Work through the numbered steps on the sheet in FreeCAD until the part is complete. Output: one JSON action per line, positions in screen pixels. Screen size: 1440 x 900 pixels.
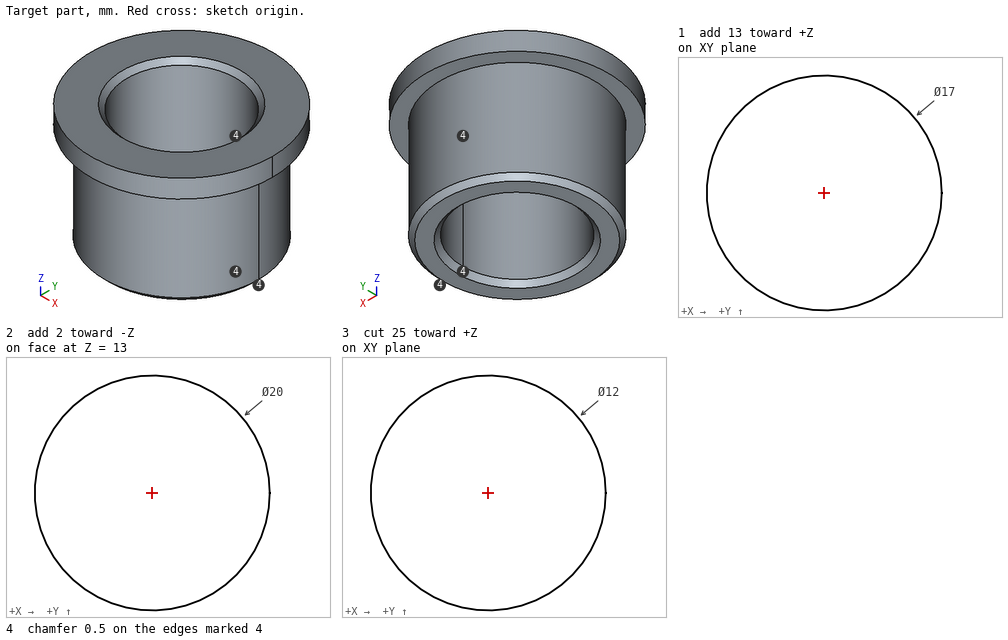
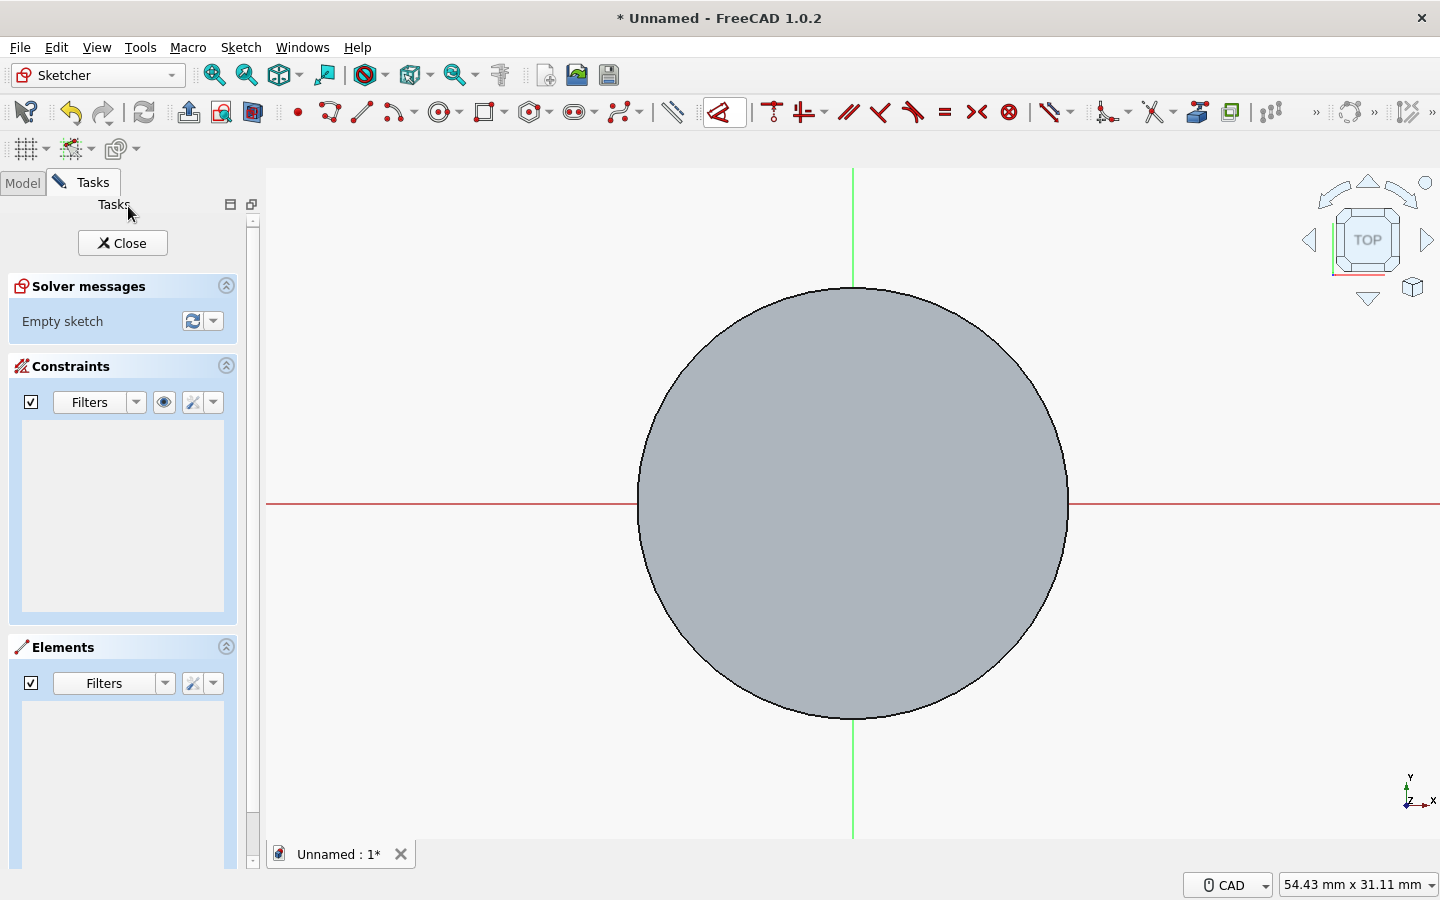
{"action": "key", "text": "q s"}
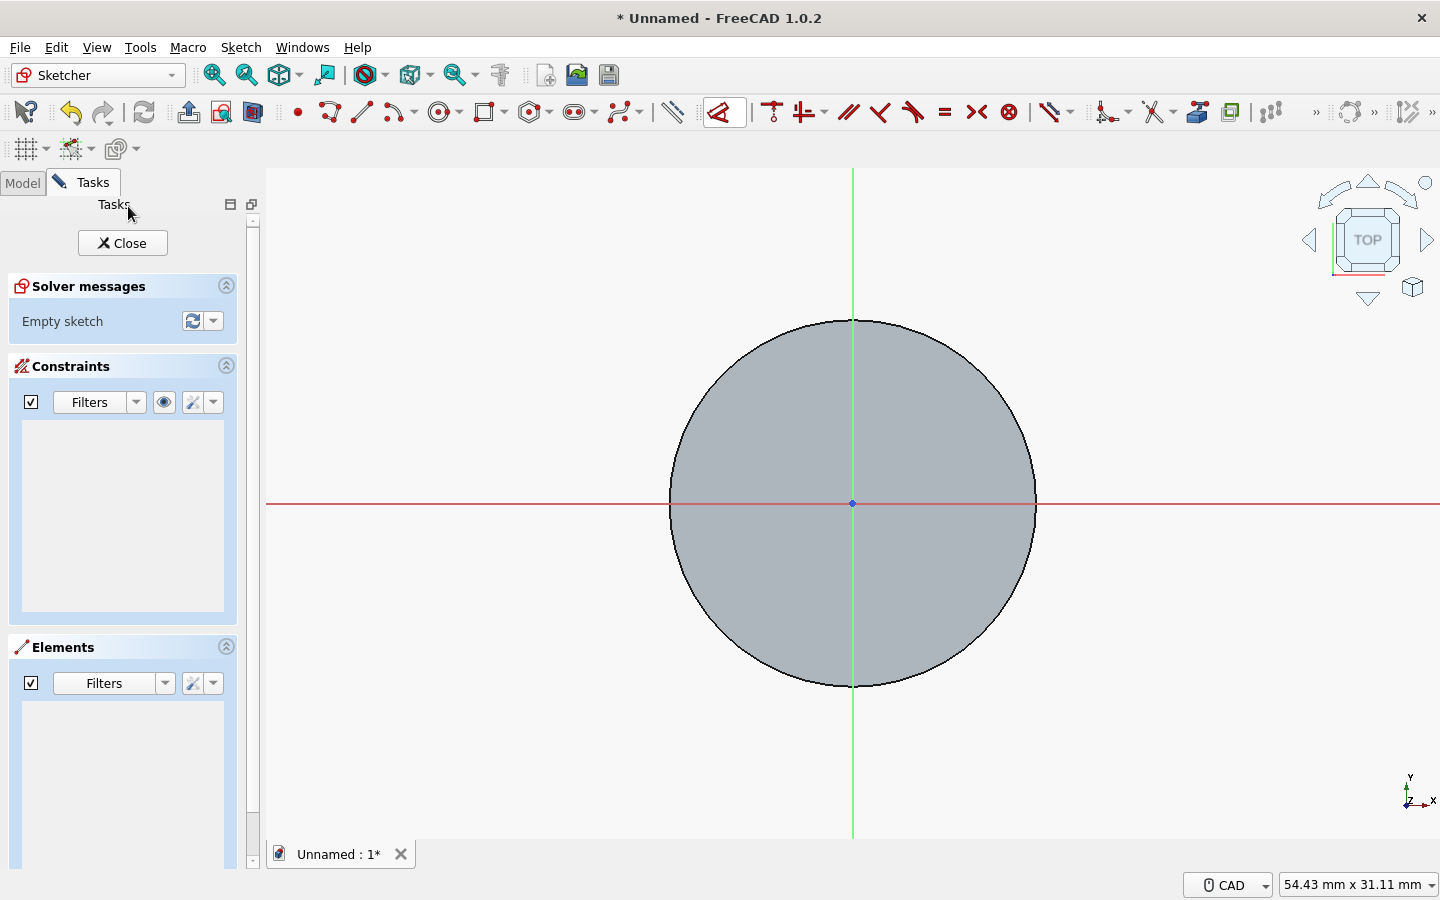
{"action": "scroll", "coordinate": [936, 504], "scroll_direction": "up", "scroll_amount": 3}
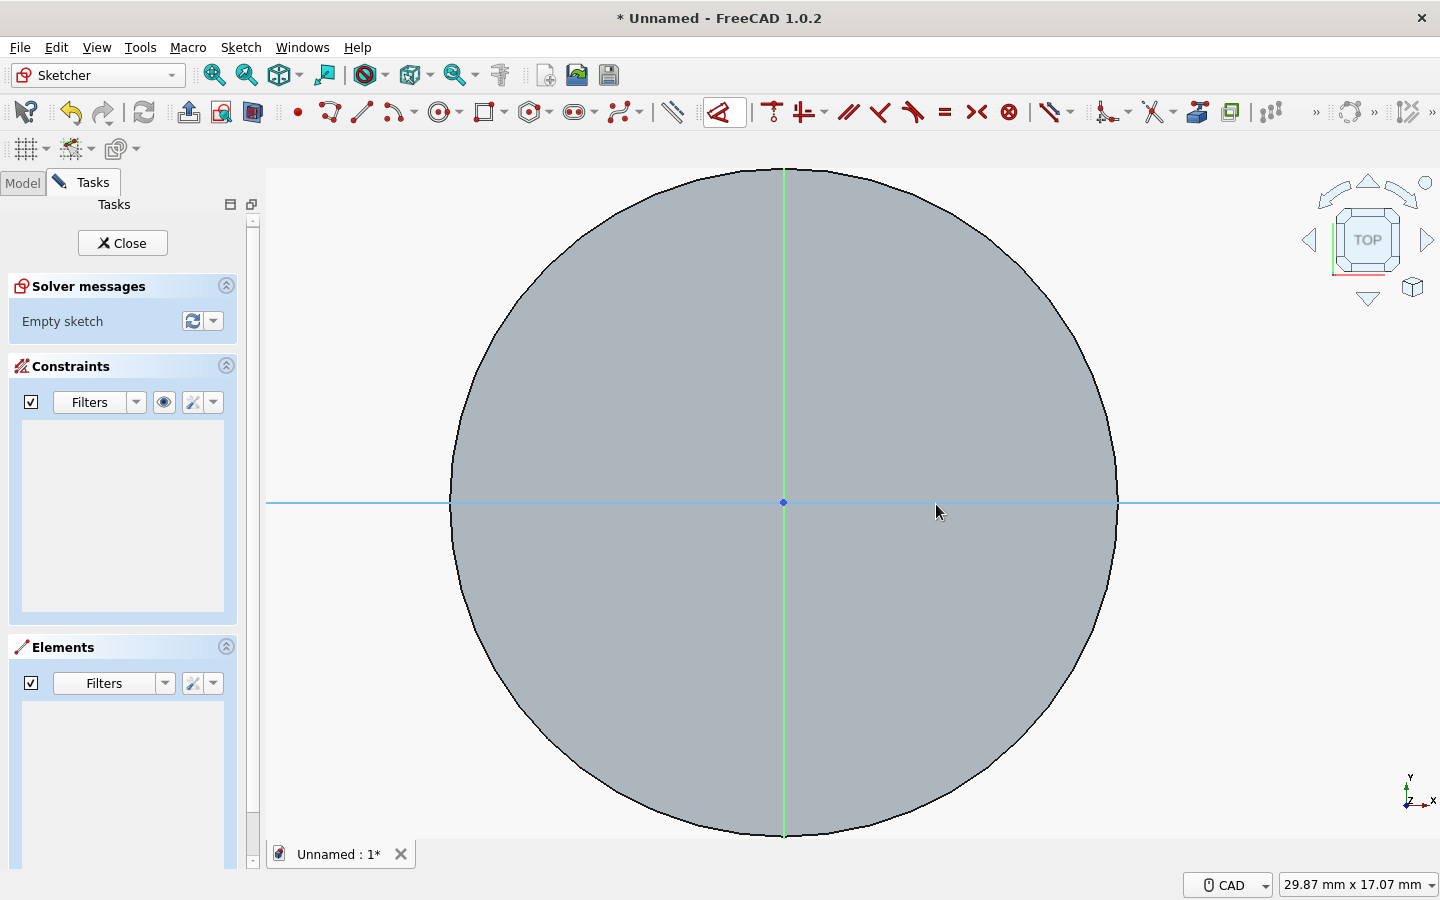
{"action": "key", "text": "g c"}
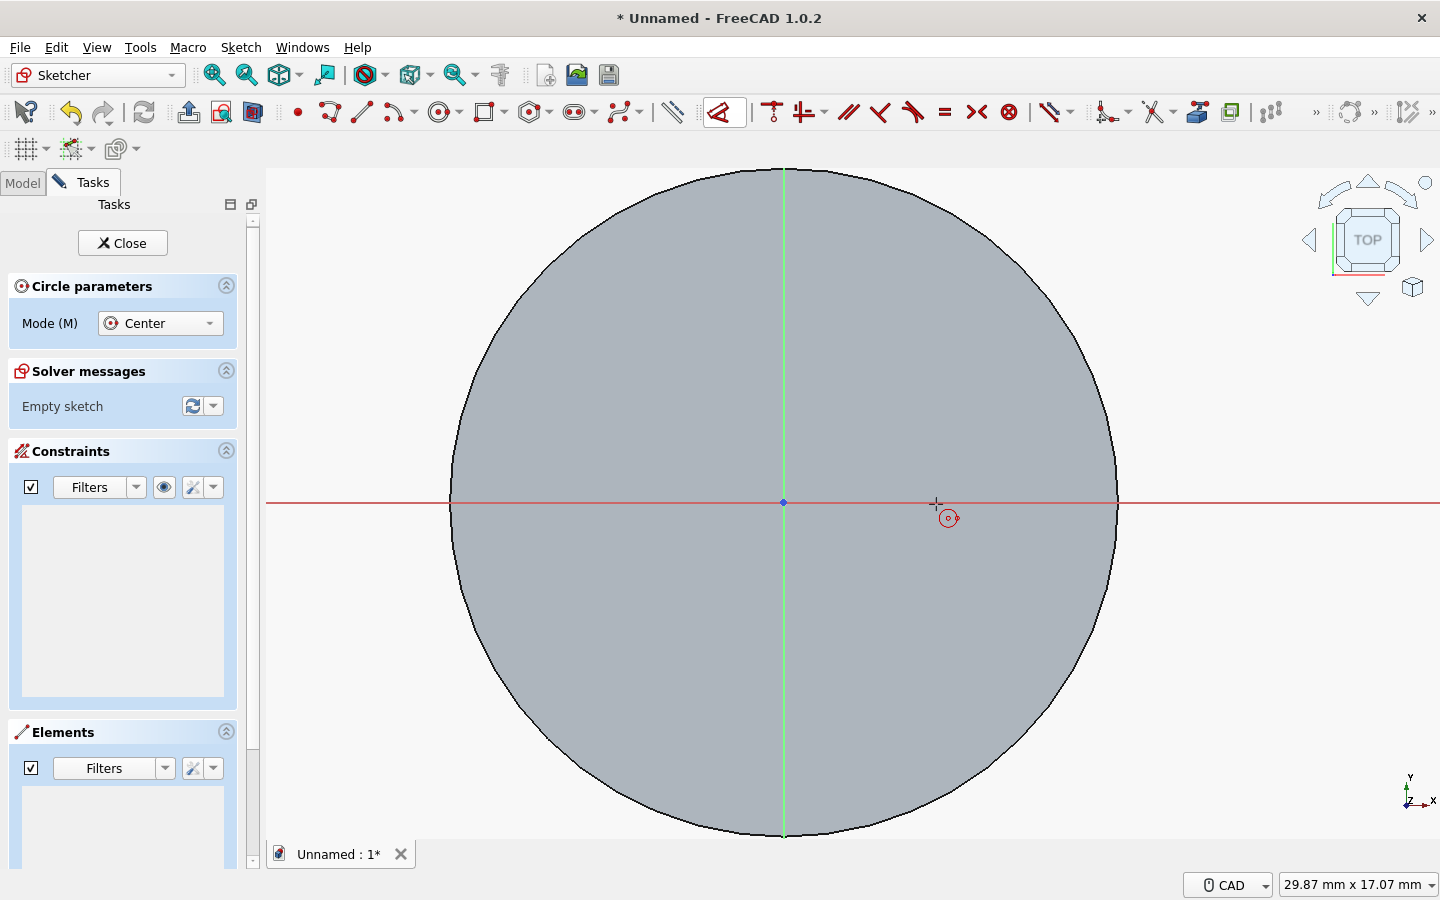
{"action": "left_click", "coordinate": [784, 503]}
{"action": "left_click", "coordinate": [951, 336]}
{"action": "key", "text": "Escape"}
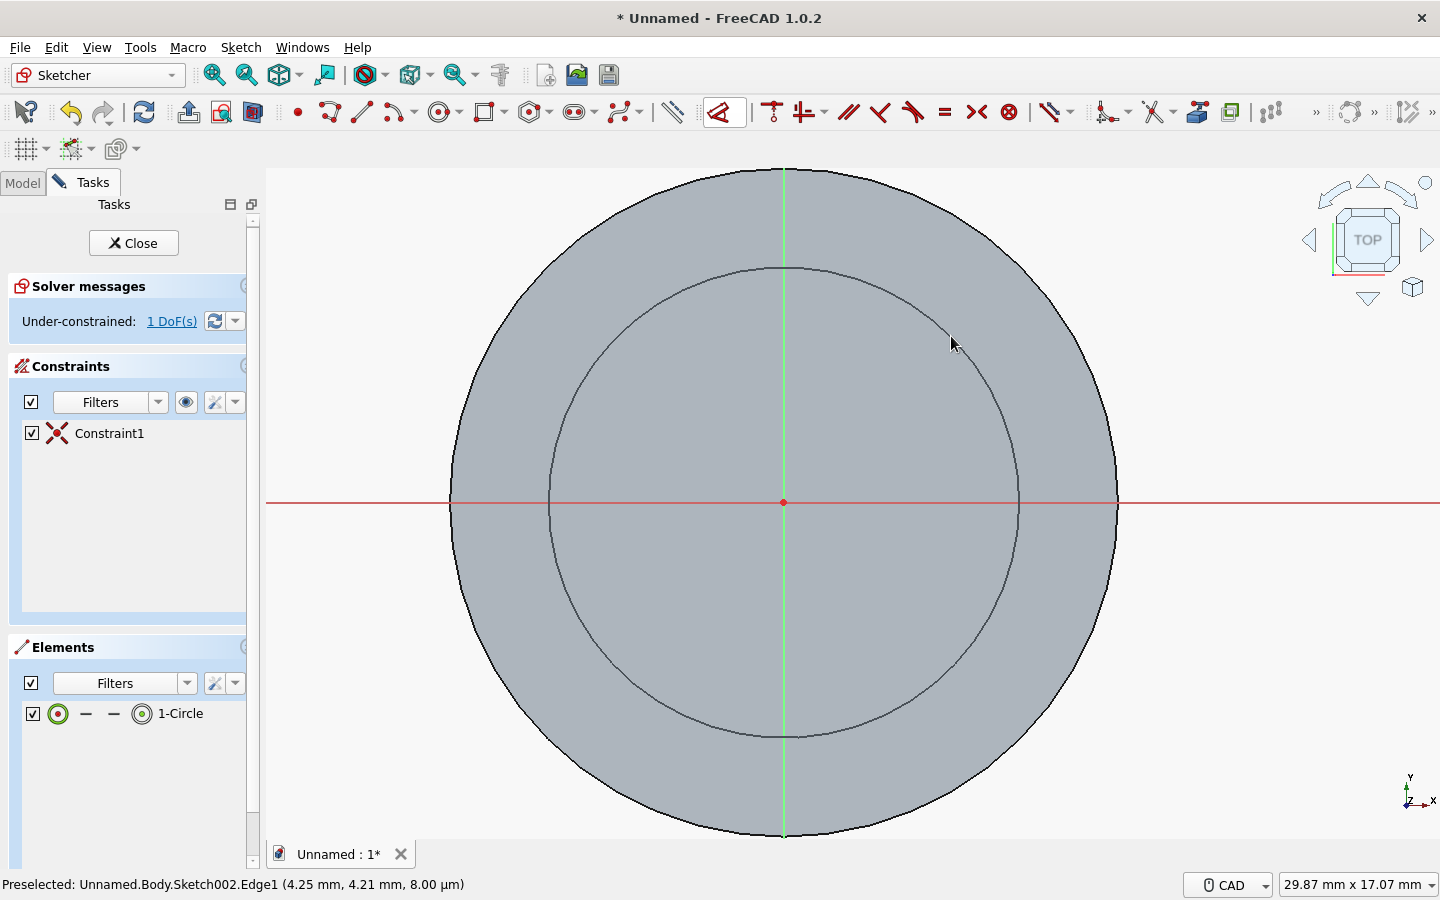
{"action": "left_click", "coordinate": [950, 336]}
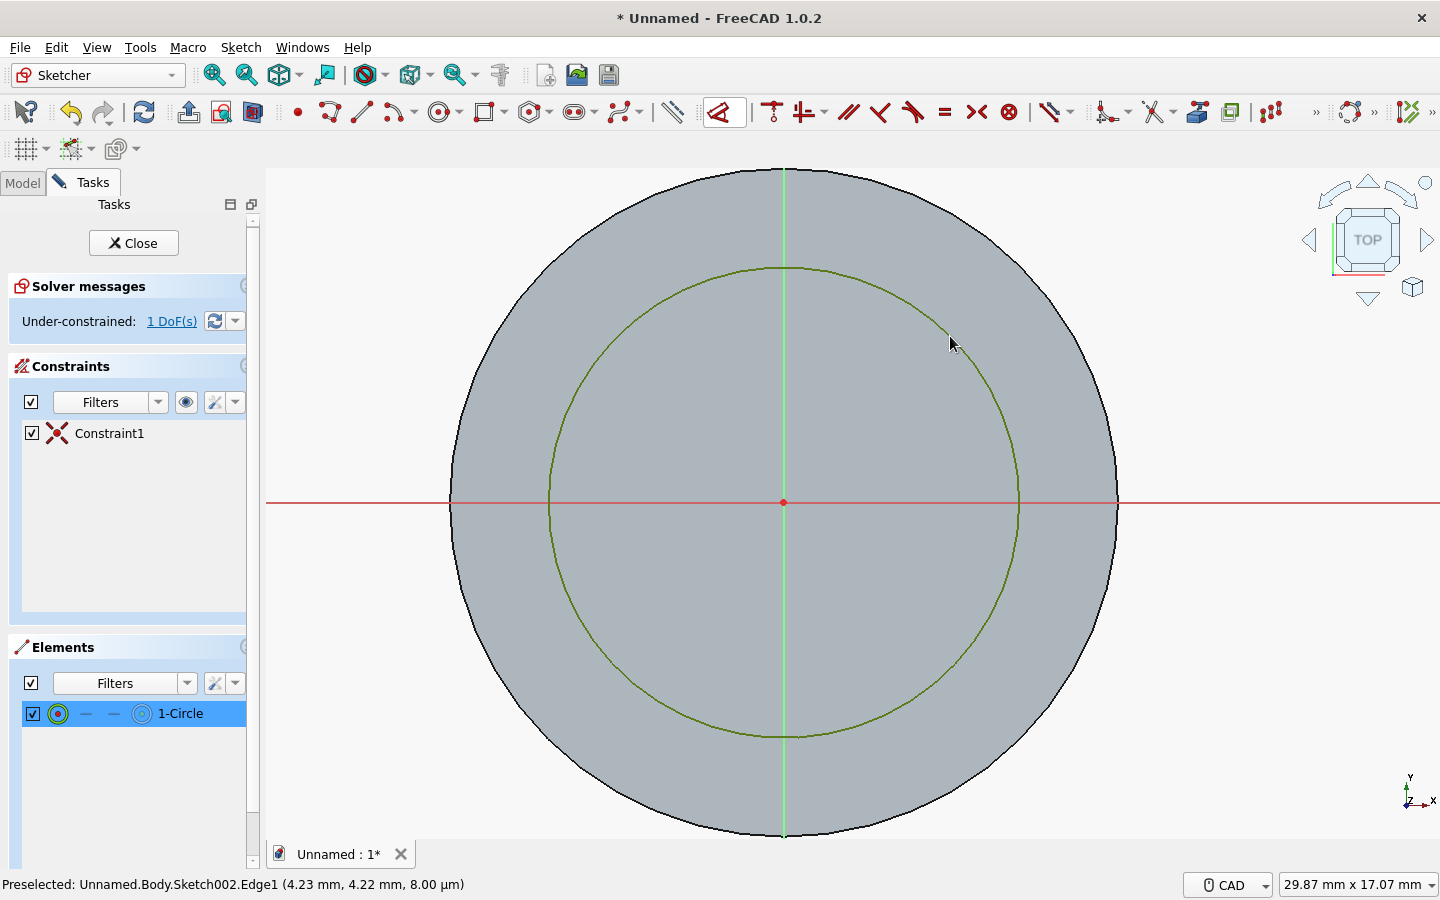
{"action": "key", "text": "k o"}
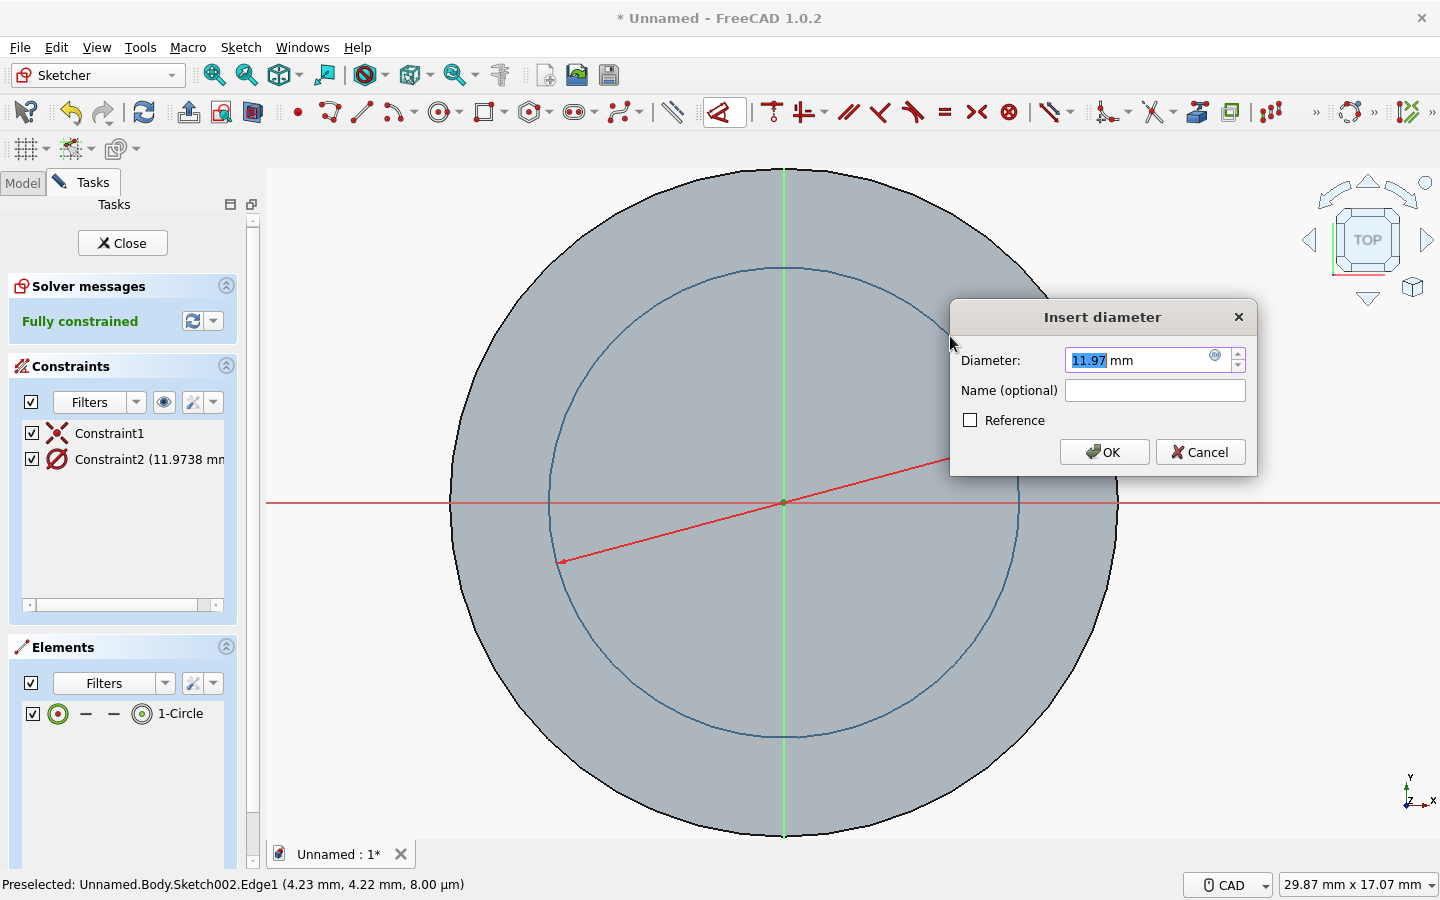
{"action": "type", "text": "12"}
{"action": "key", "text": "Return"}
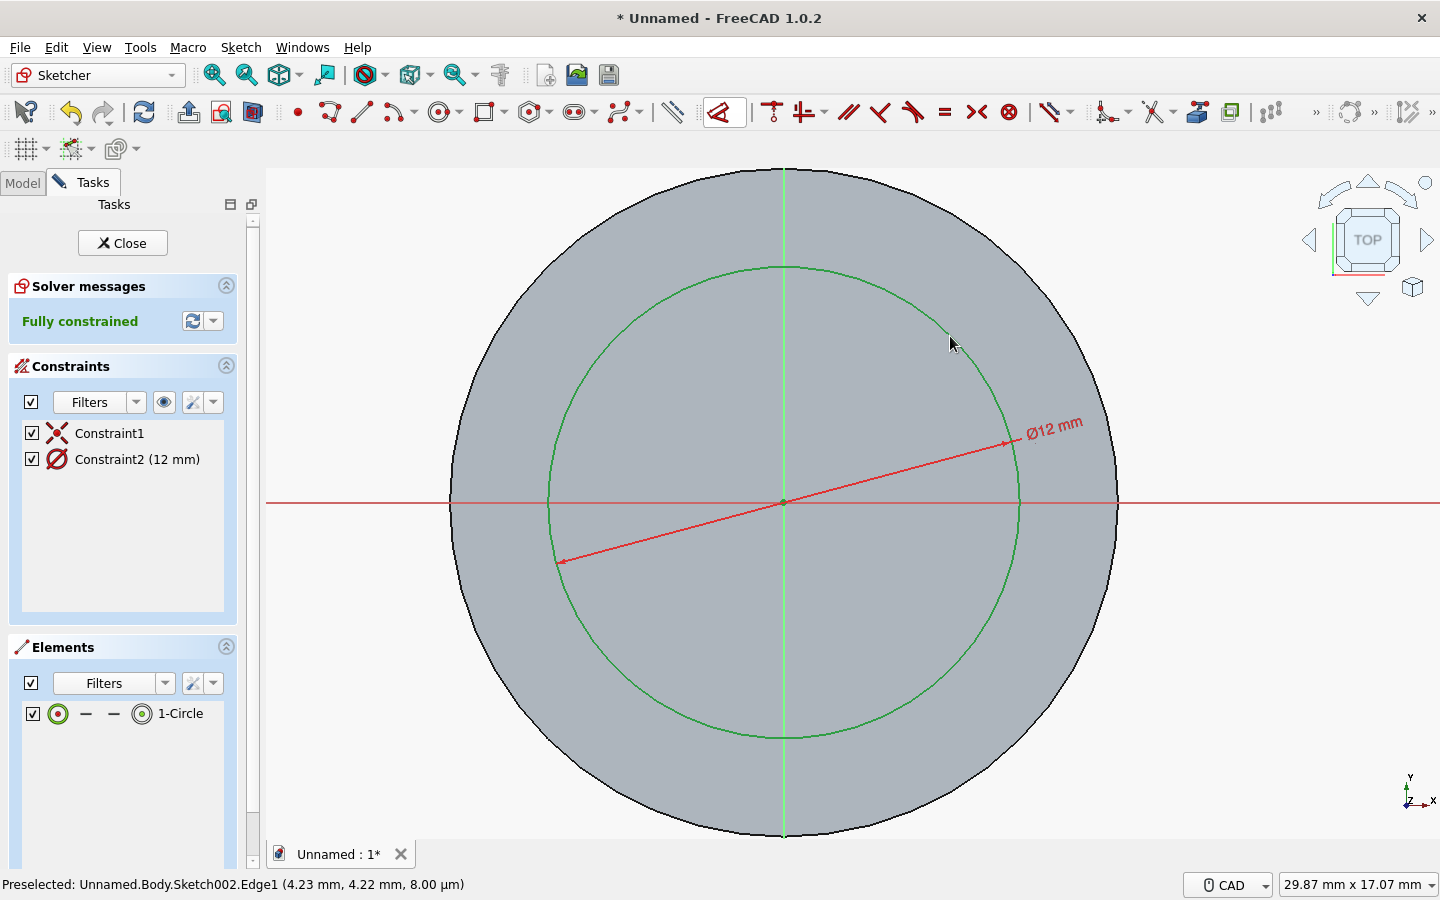
{"action": "left_click", "coordinate": [123, 243]}